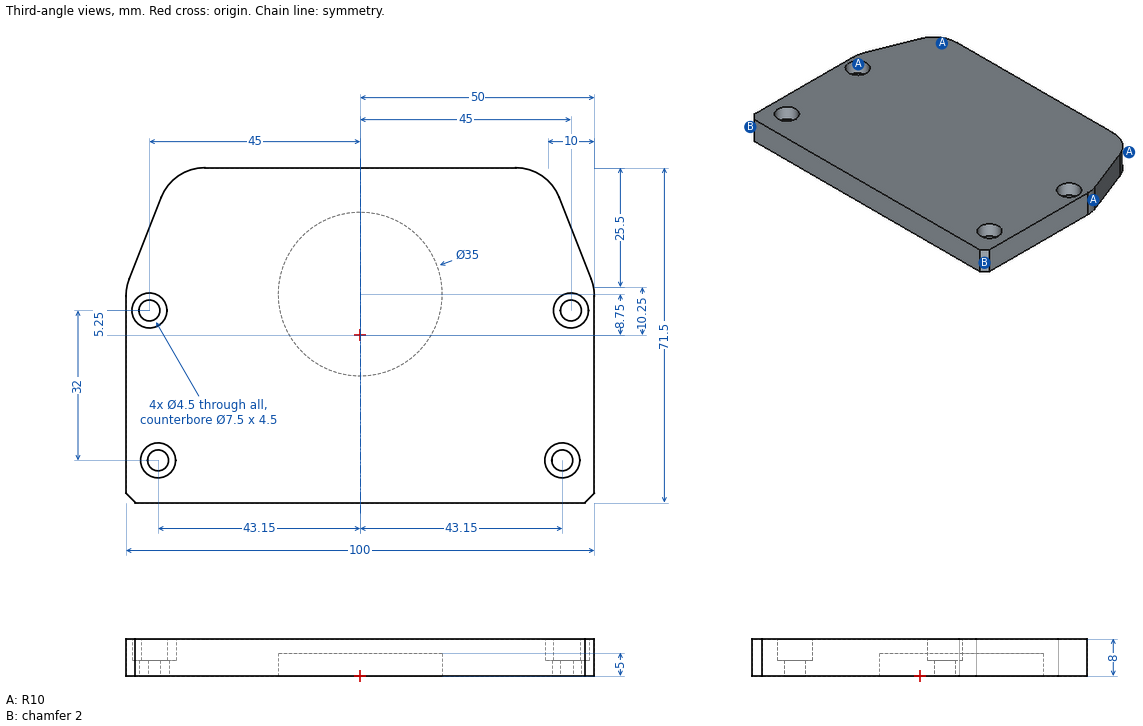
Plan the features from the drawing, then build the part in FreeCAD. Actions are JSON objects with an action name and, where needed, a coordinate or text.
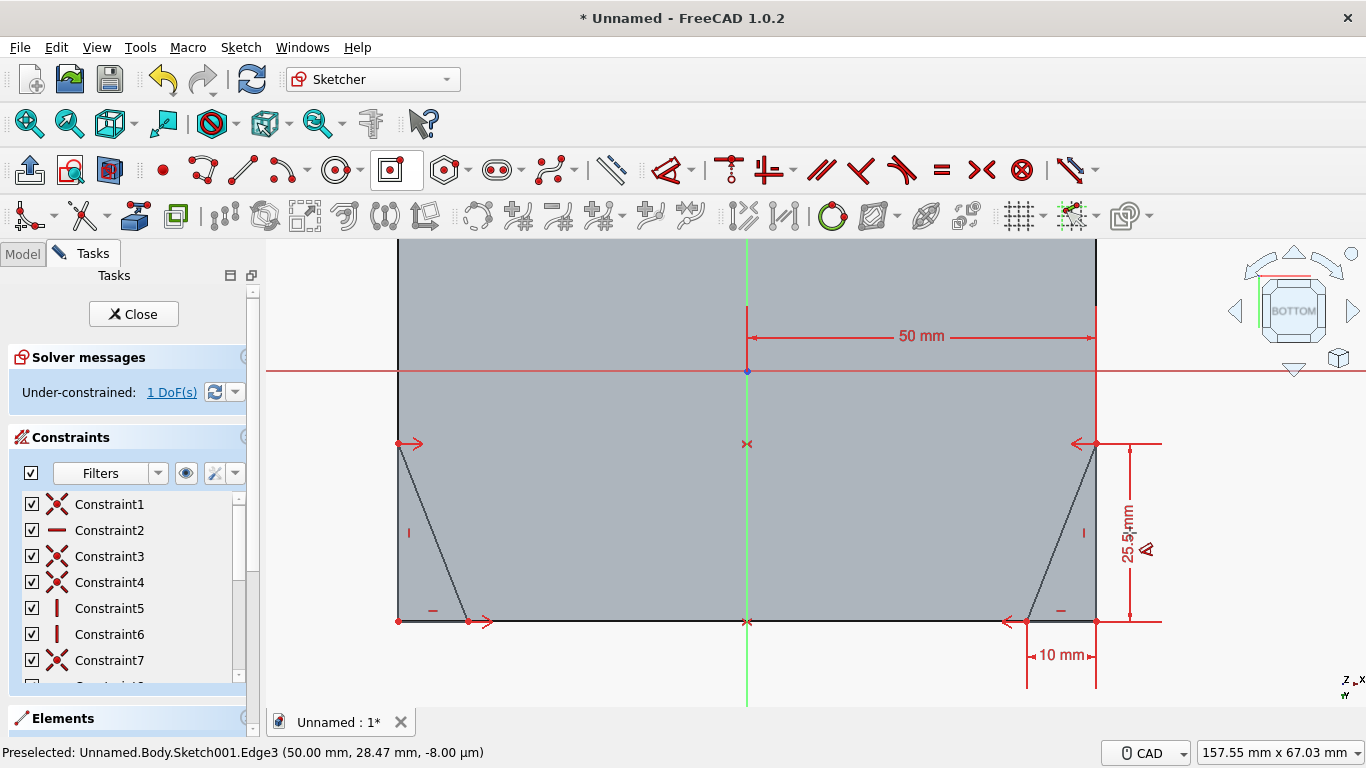
{"action": "left_click", "coordinate": [1096, 444]}
{"action": "left_click", "coordinate": [1130, 408]}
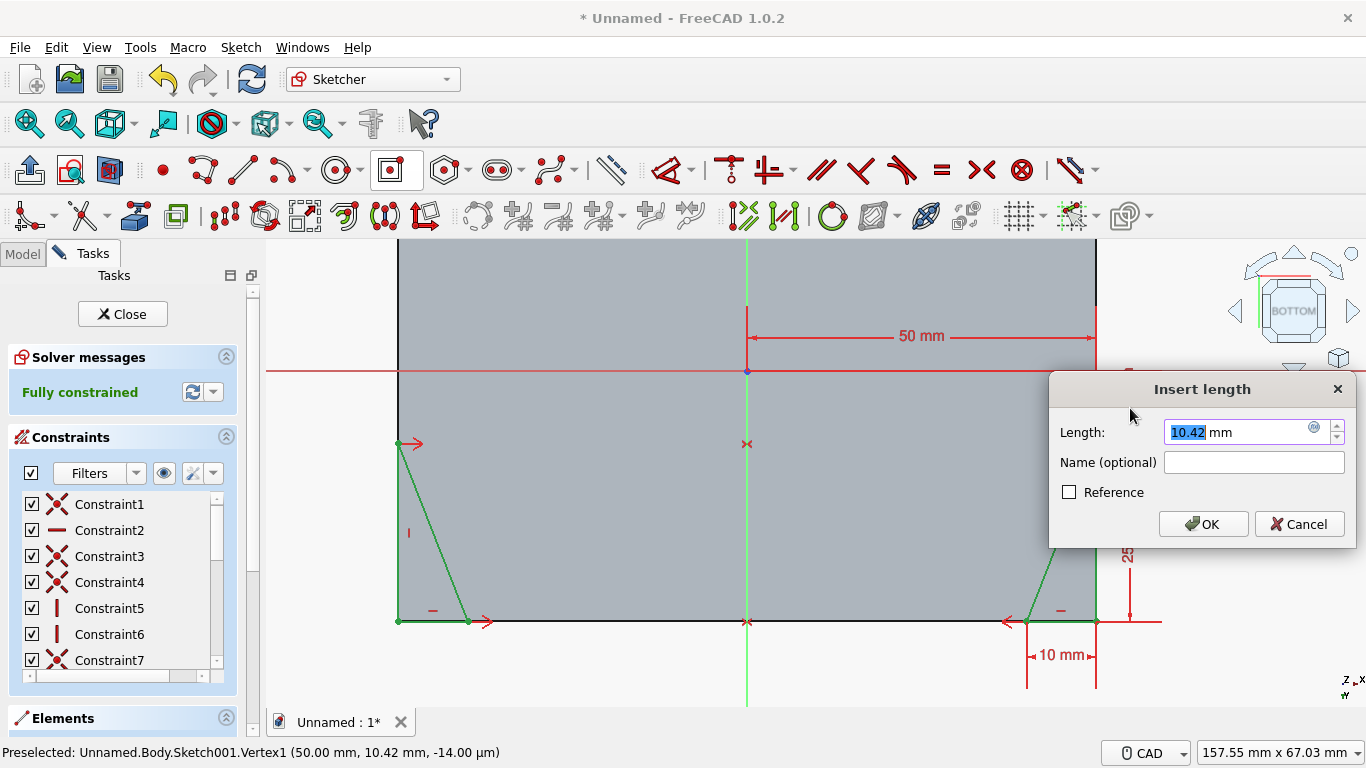
{"action": "type", "text": "10.25"}
{"action": "key", "text": "Return"}
{"action": "key", "text": "Escape"}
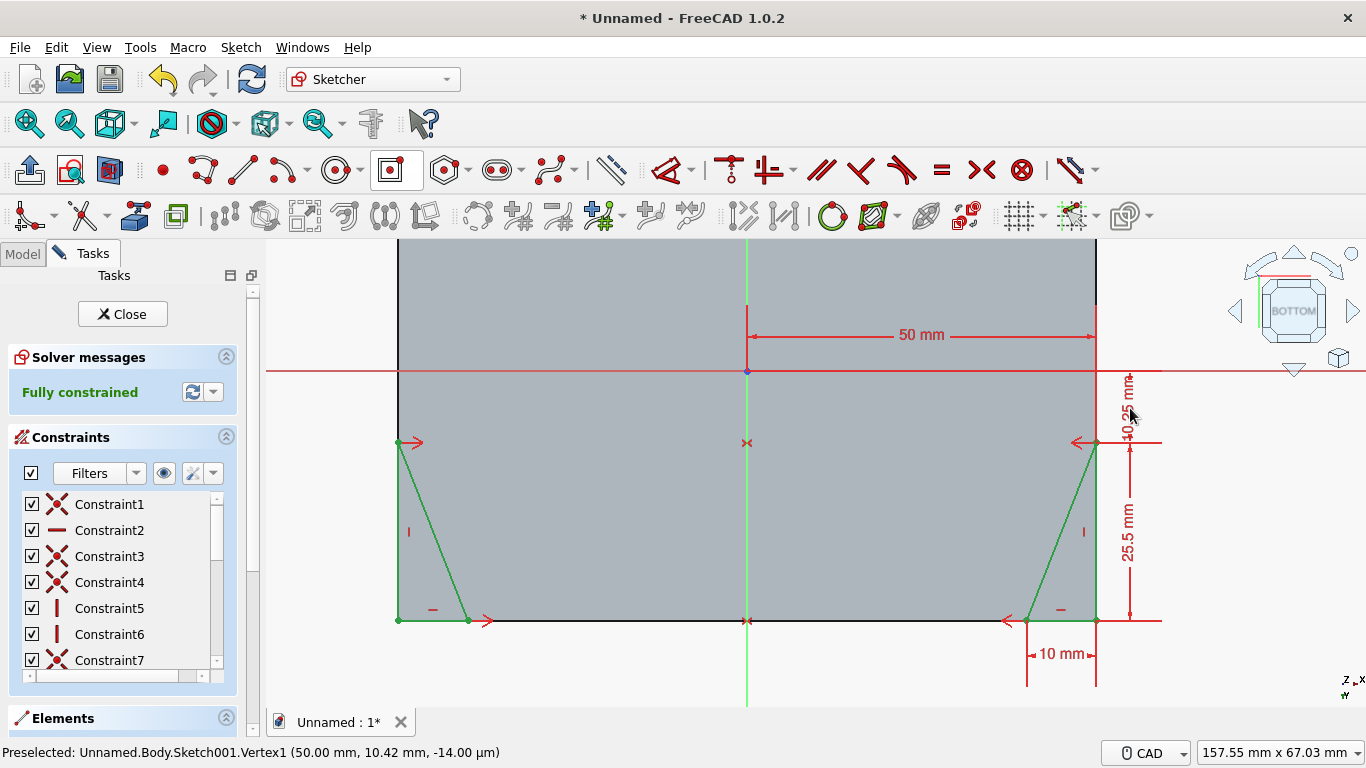
{"action": "left_click", "coordinate": [123, 314]}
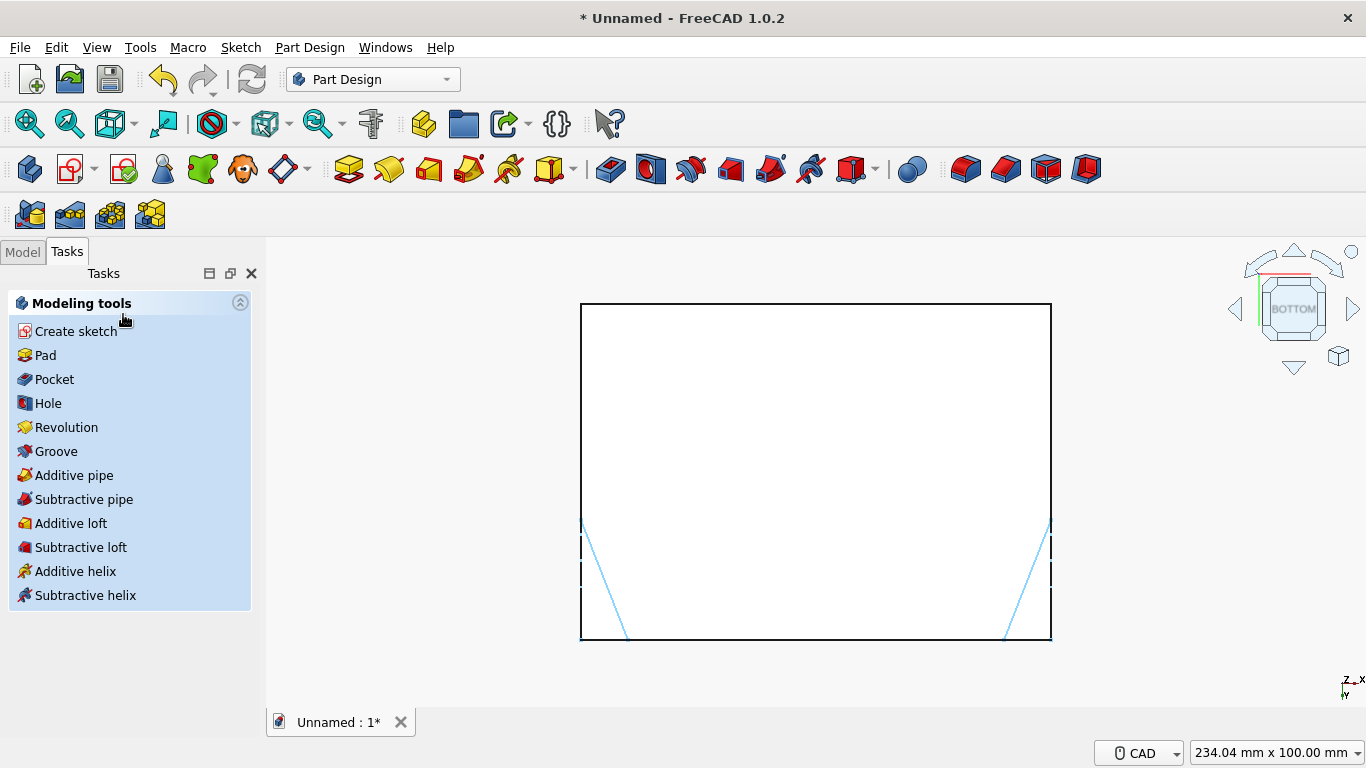
{"action": "left_click", "coordinate": [612, 170]}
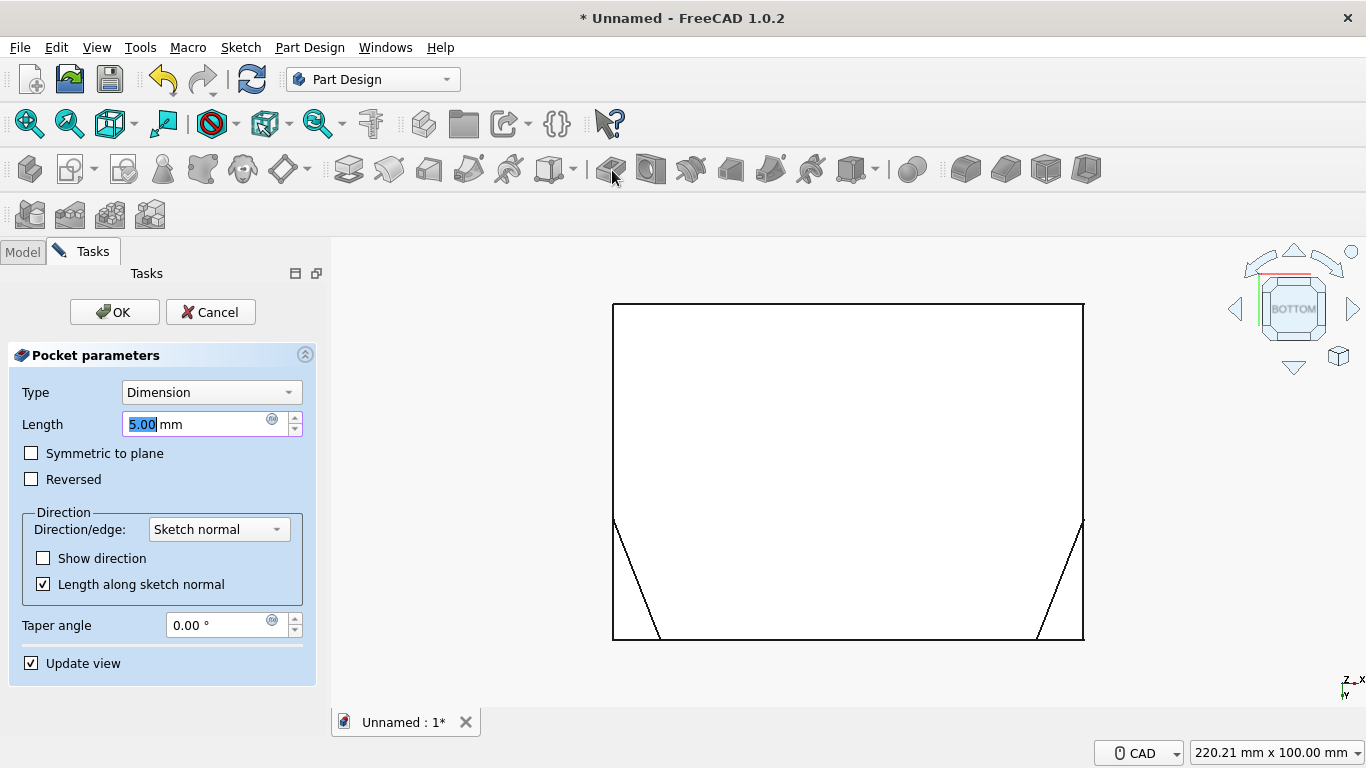
{"action": "type", "text": "10"}
{"action": "key", "text": "Tab"}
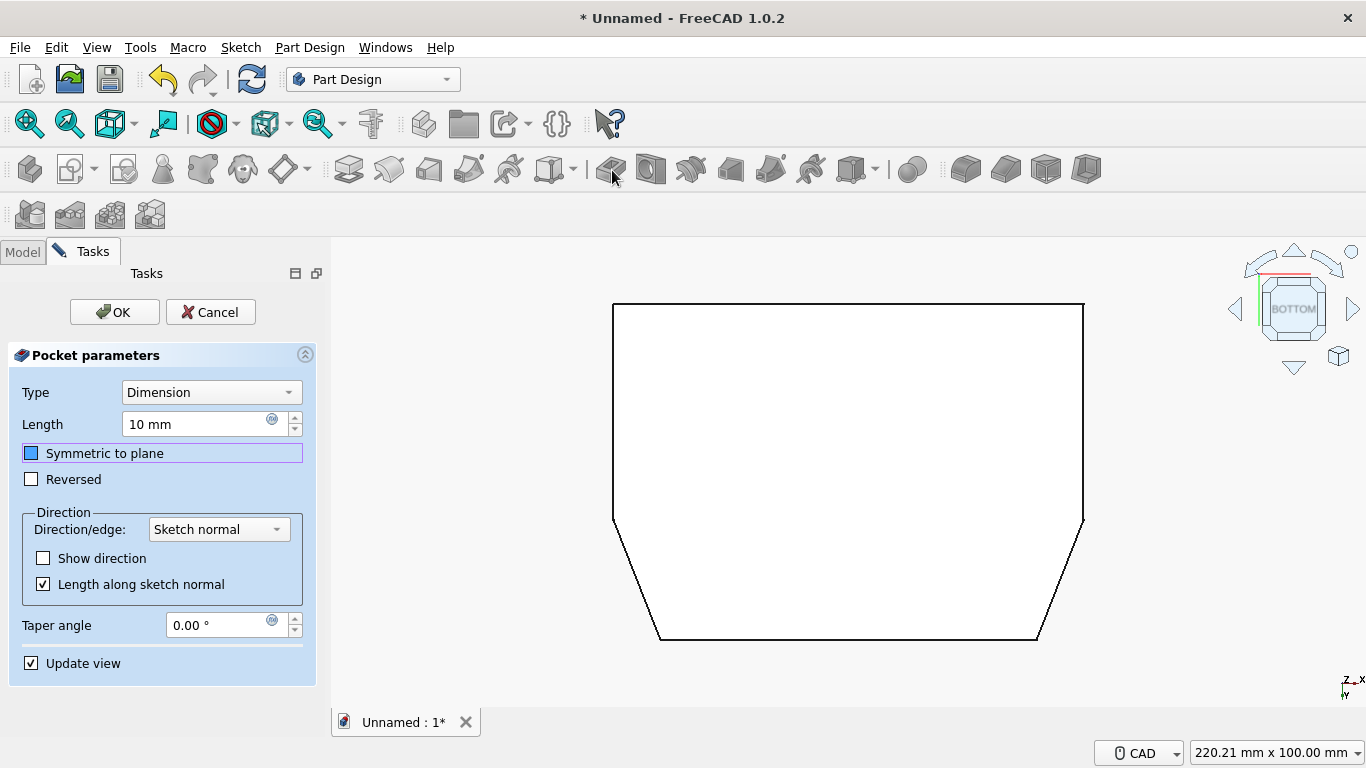
{"action": "left_click", "coordinate": [115, 312]}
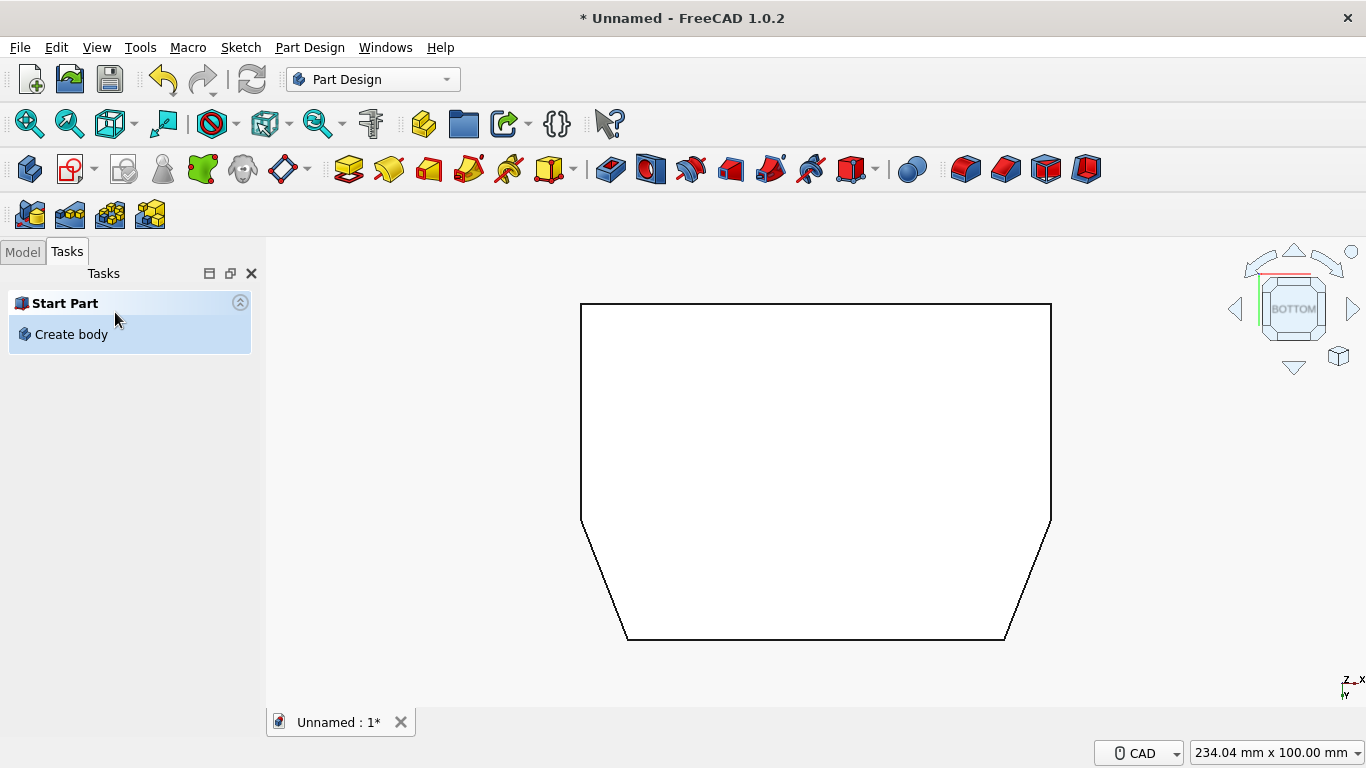
{"action": "key", "text": "0"}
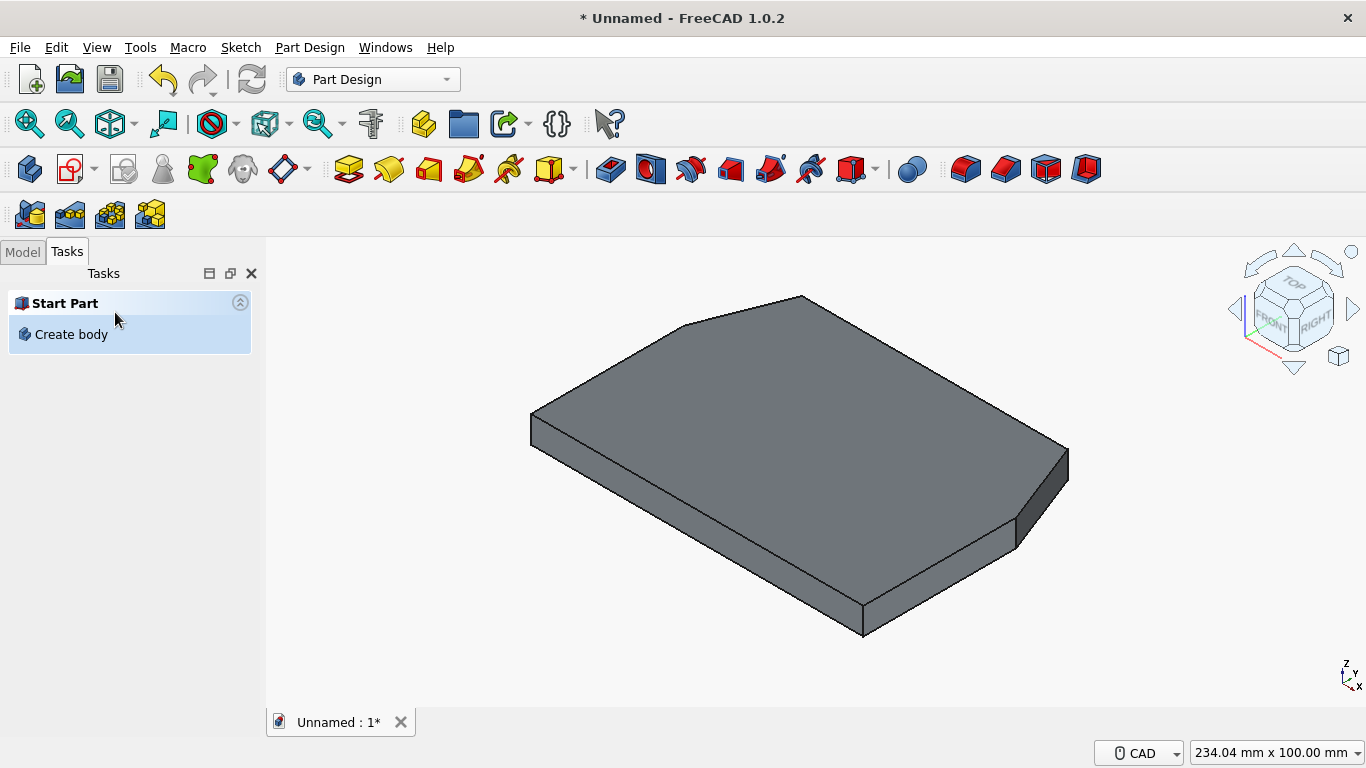
{"action": "key", "text": "2"}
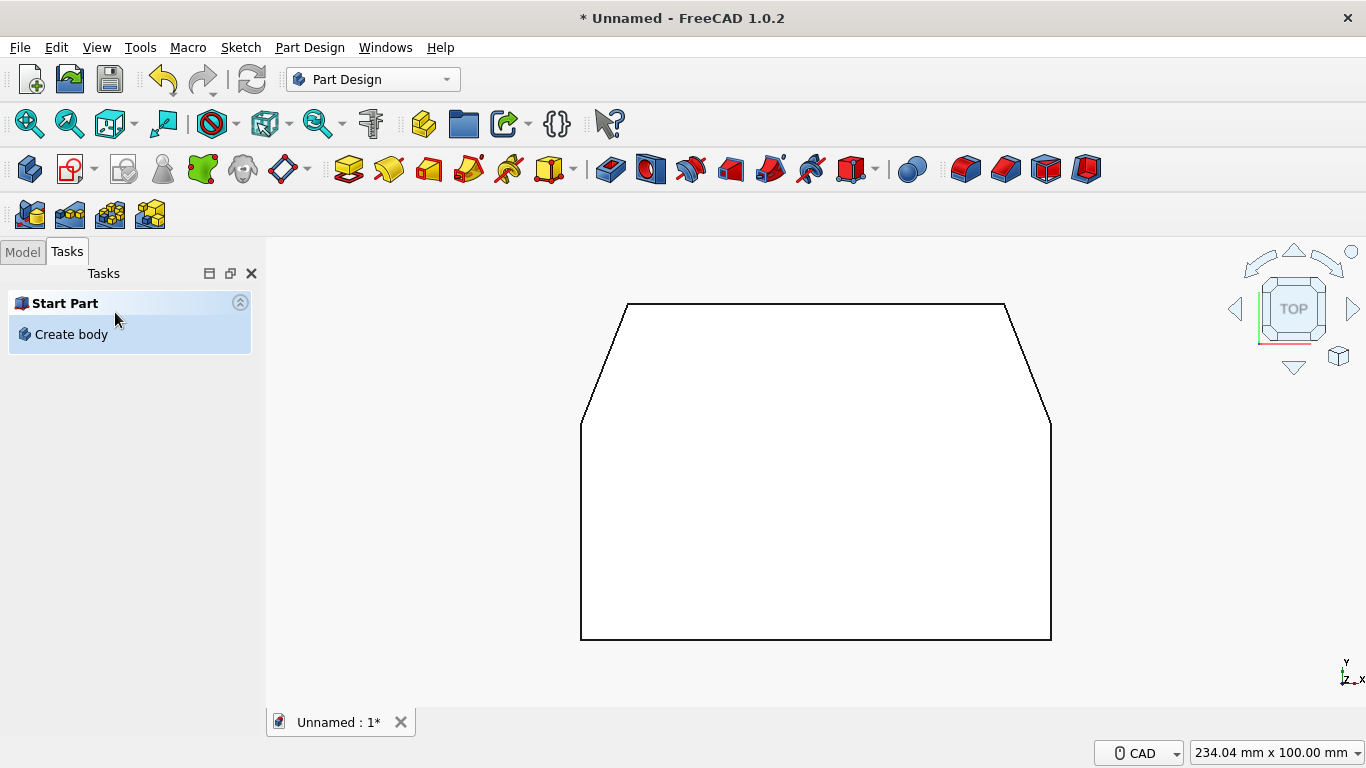
{"action": "key", "text": "1"}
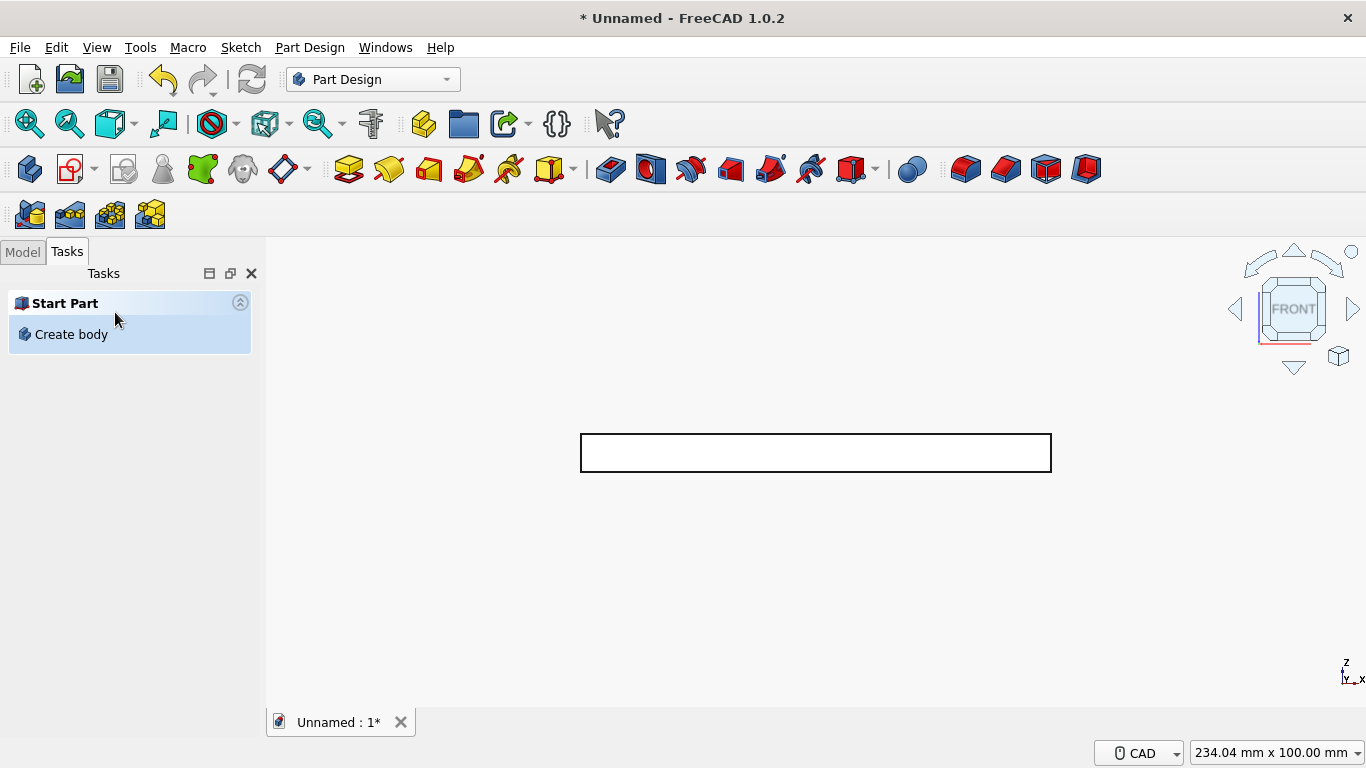
{"action": "left_click", "coordinate": [30, 124]}